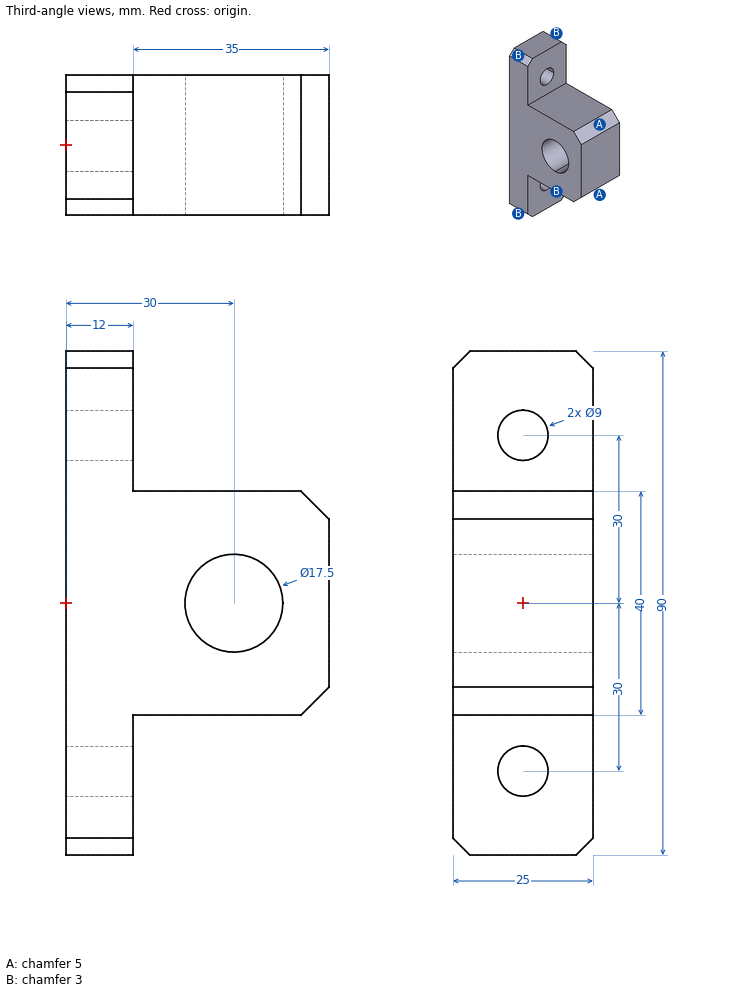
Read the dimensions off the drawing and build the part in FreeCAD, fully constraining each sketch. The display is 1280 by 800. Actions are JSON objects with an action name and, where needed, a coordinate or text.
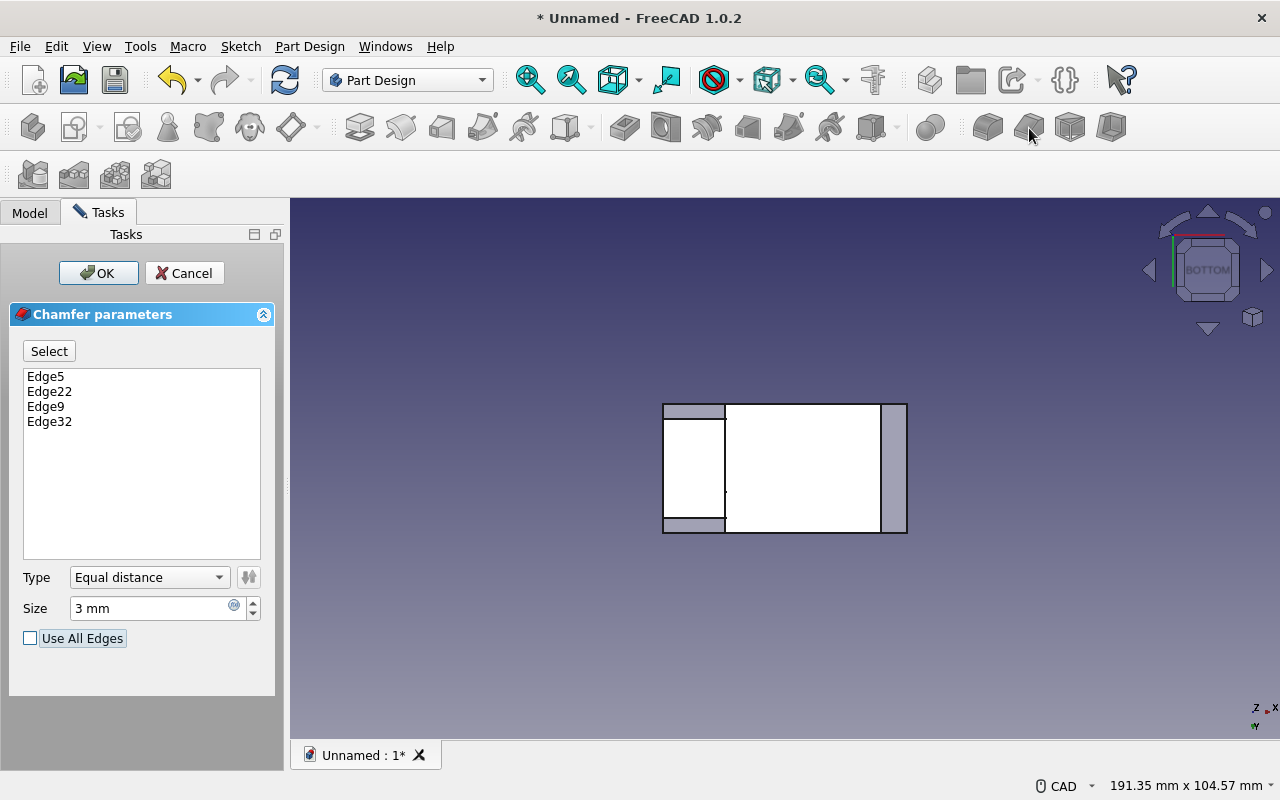
{"action": "left_click", "coordinate": [99, 273]}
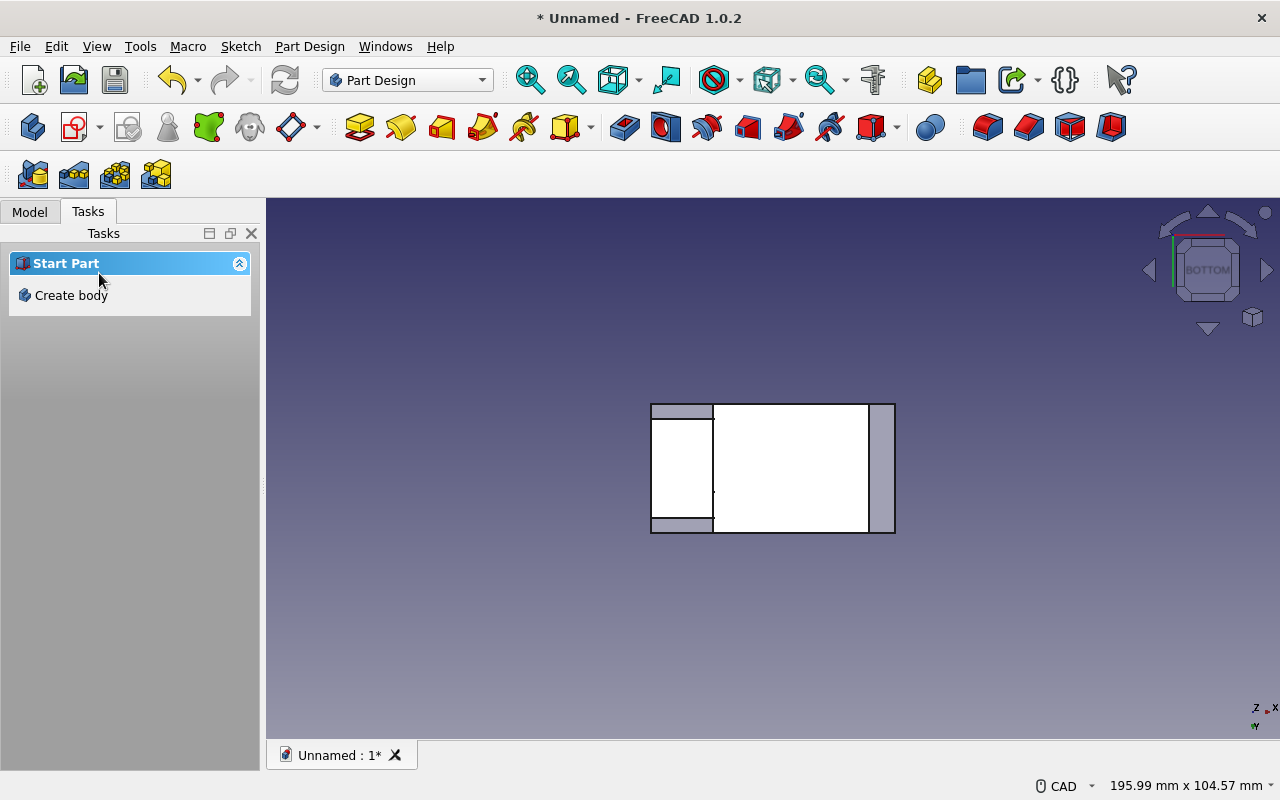
{"action": "key", "text": "0"}